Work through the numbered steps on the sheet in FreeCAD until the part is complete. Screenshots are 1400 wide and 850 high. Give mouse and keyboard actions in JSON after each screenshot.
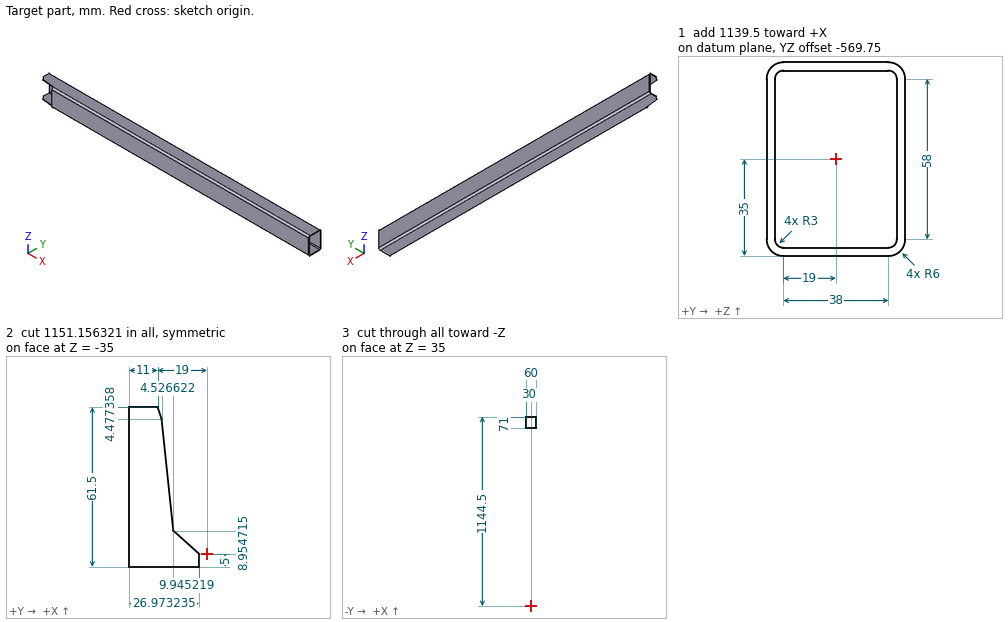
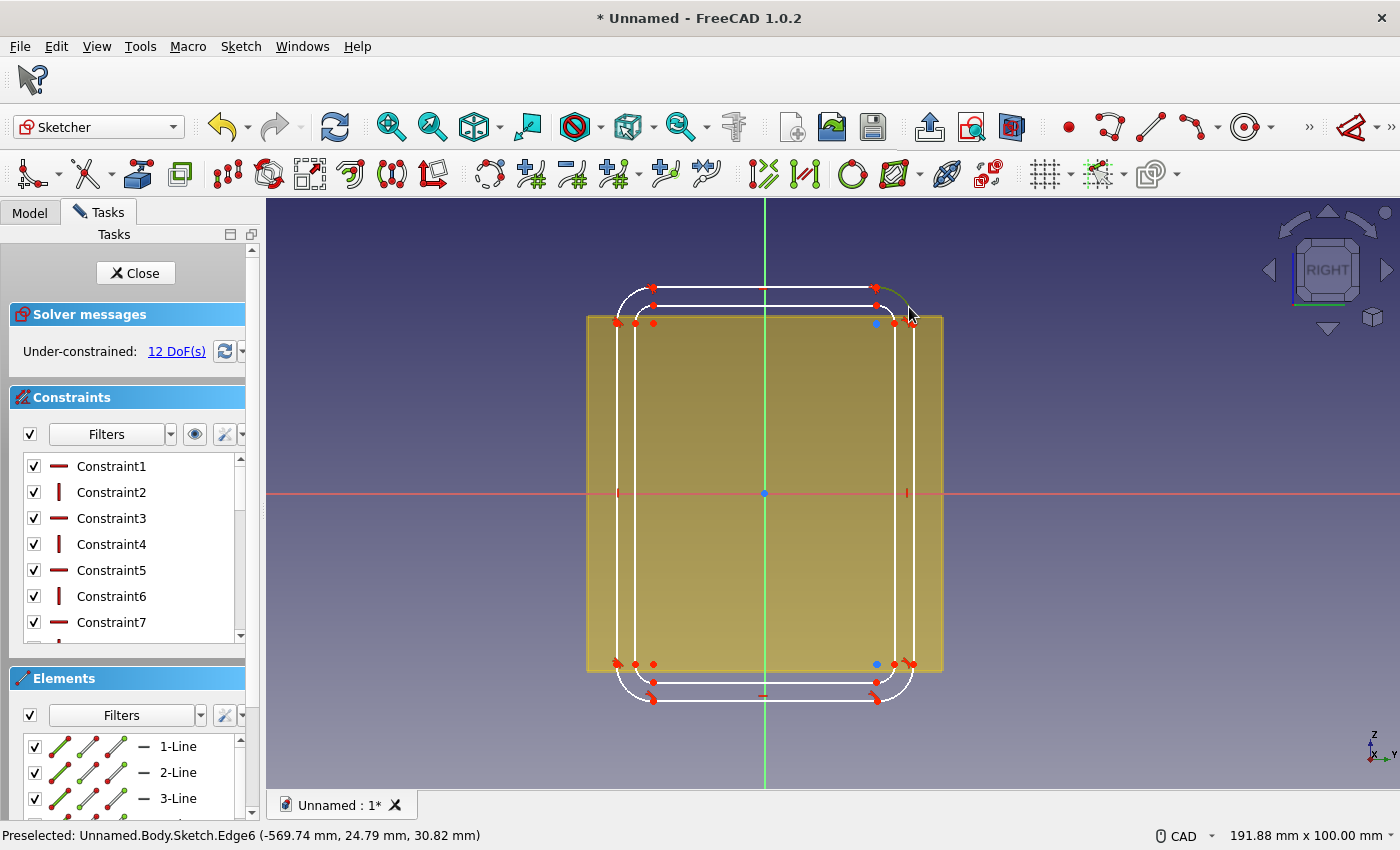
{"action": "left_click", "coordinate": [890, 311]}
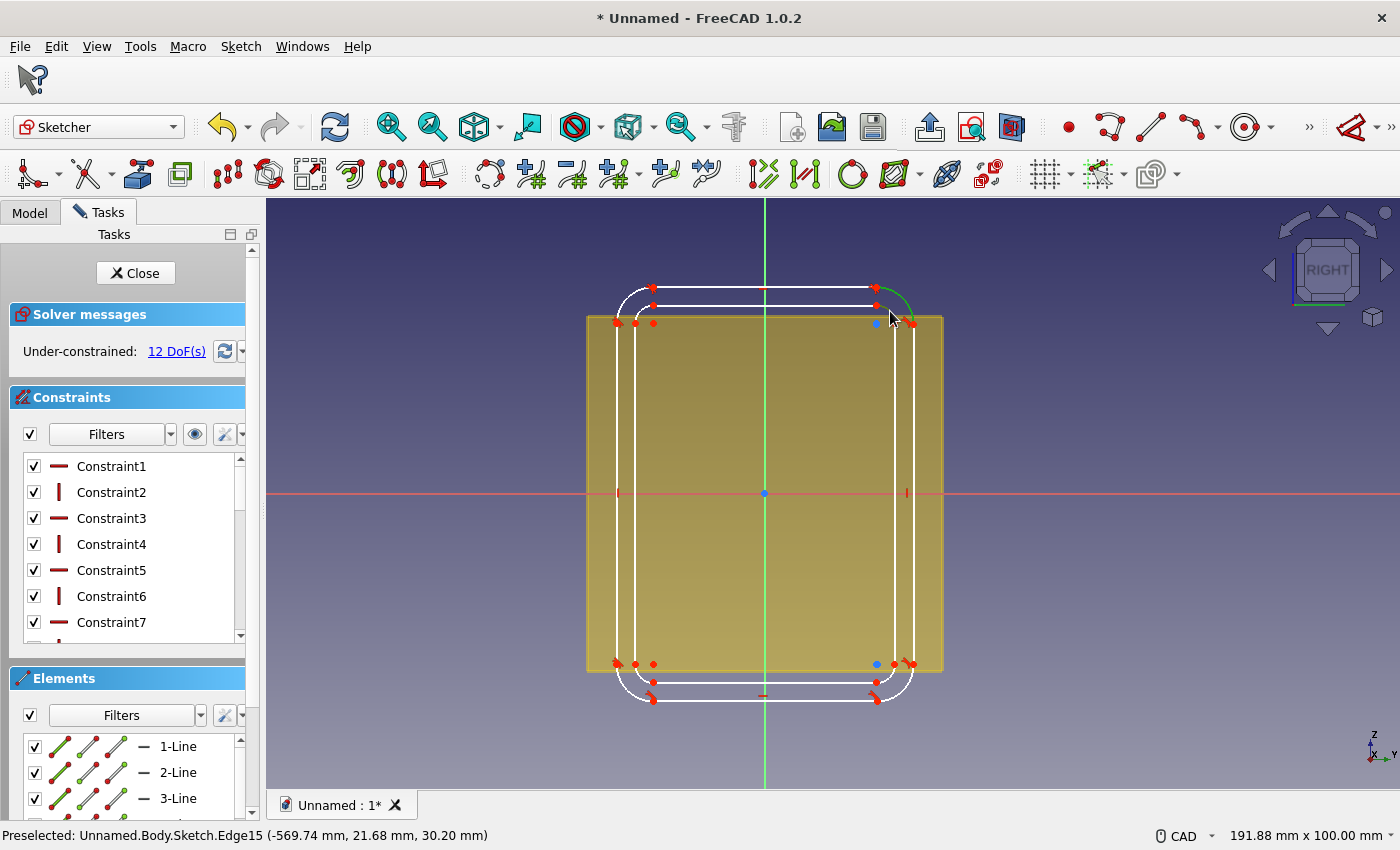
{"action": "key", "text": "c"}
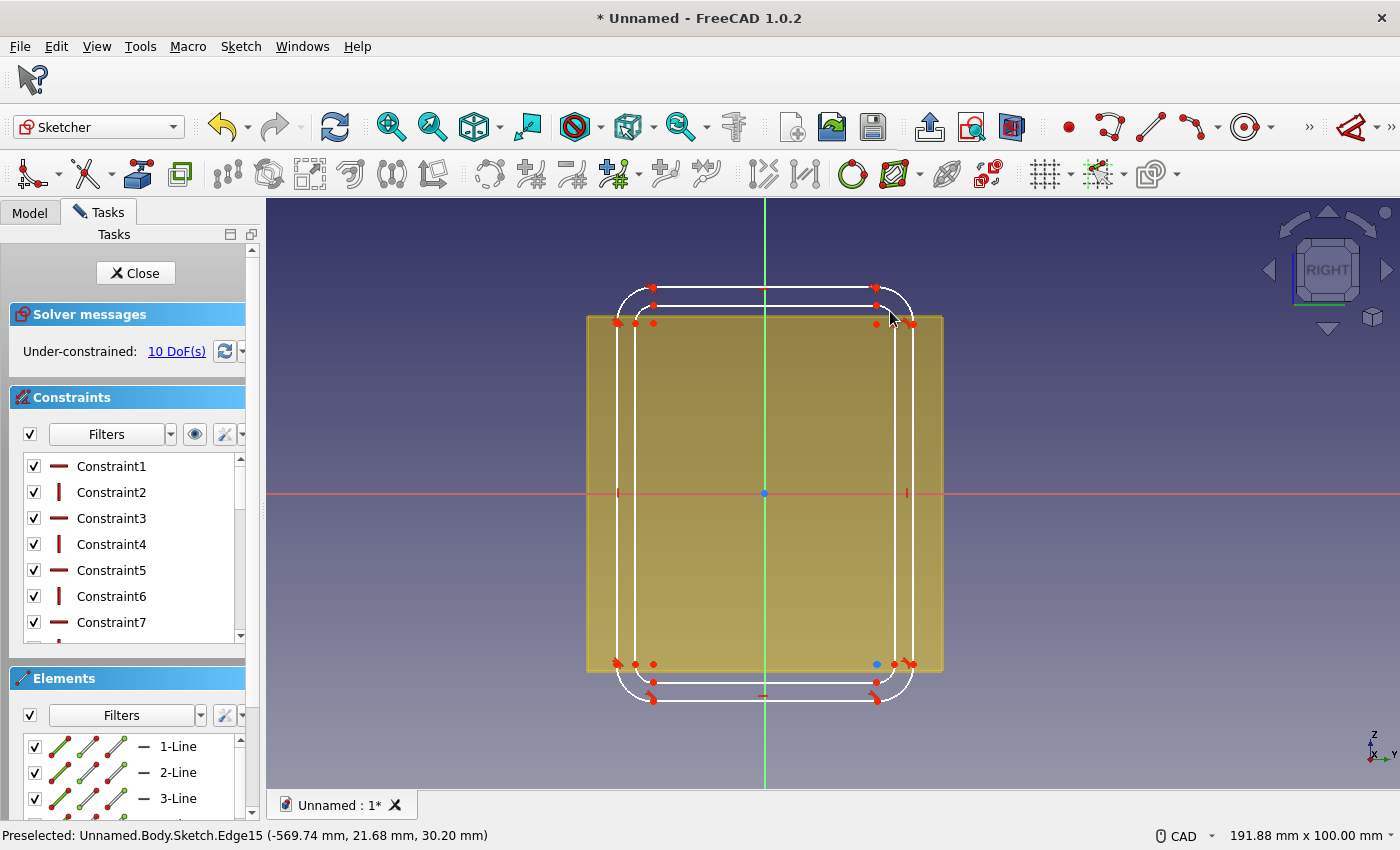
{"action": "left_click", "coordinate": [894, 697]}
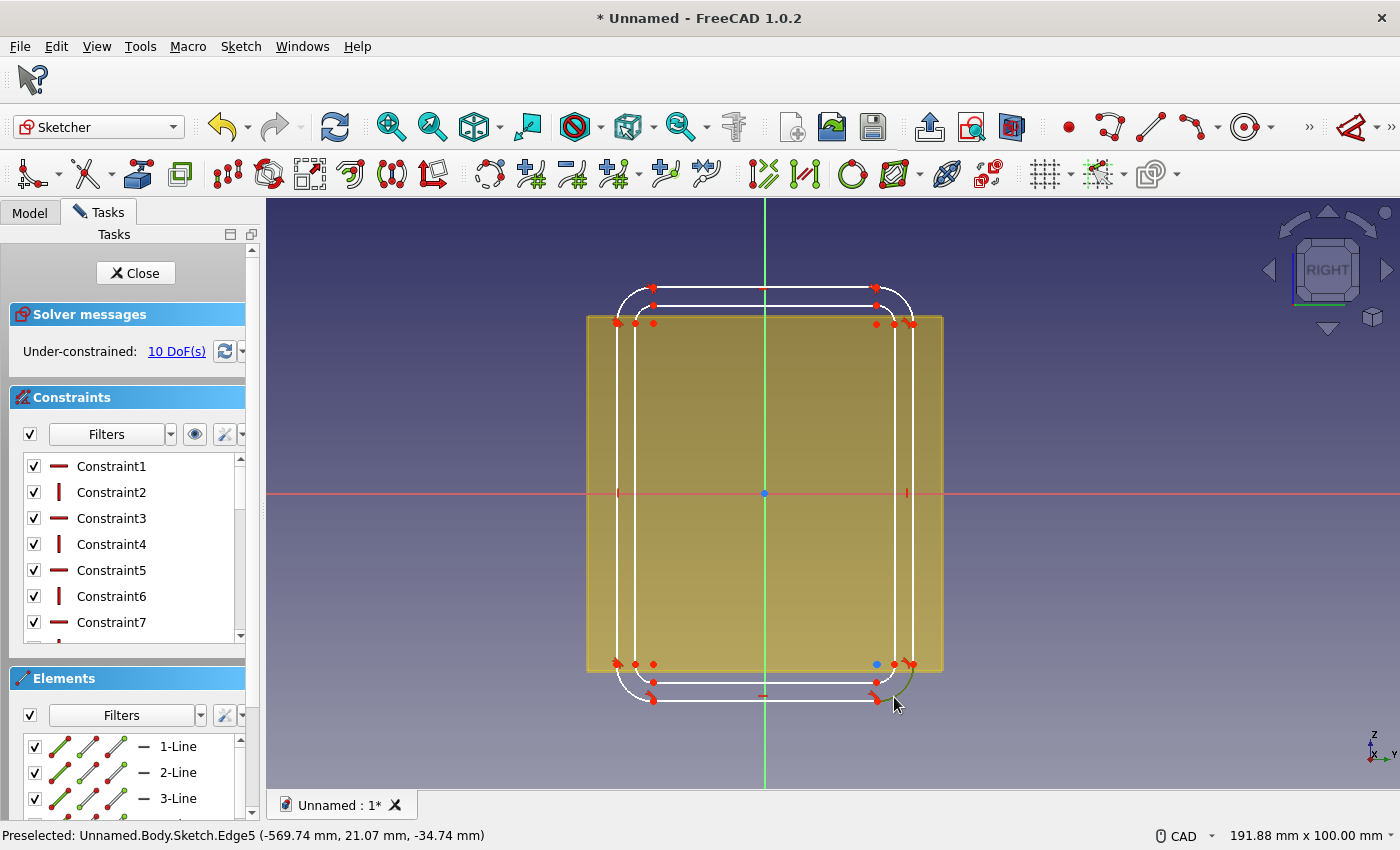
{"action": "left_click", "coordinate": [909, 307]}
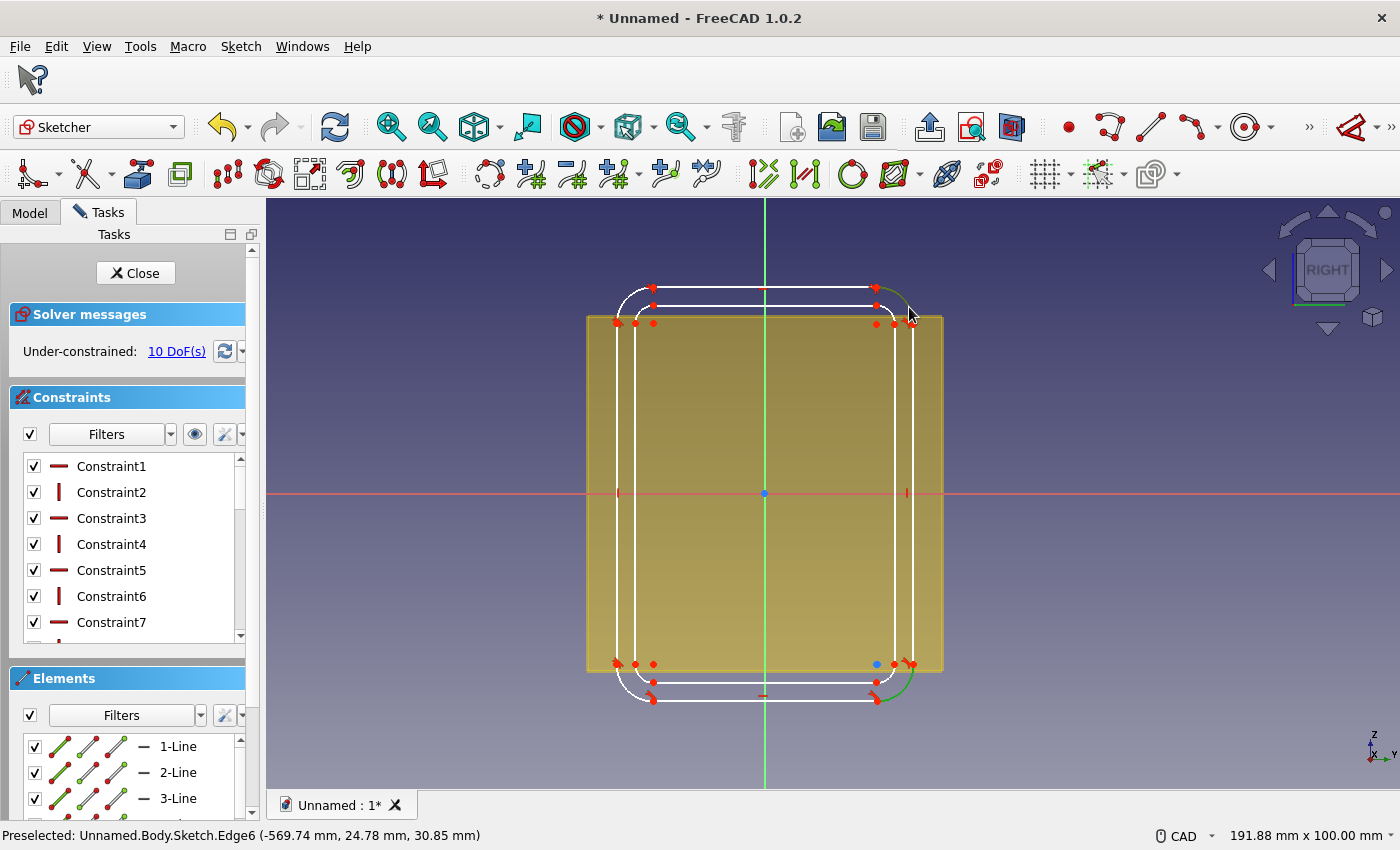
{"action": "left_click", "coordinate": [637, 291]}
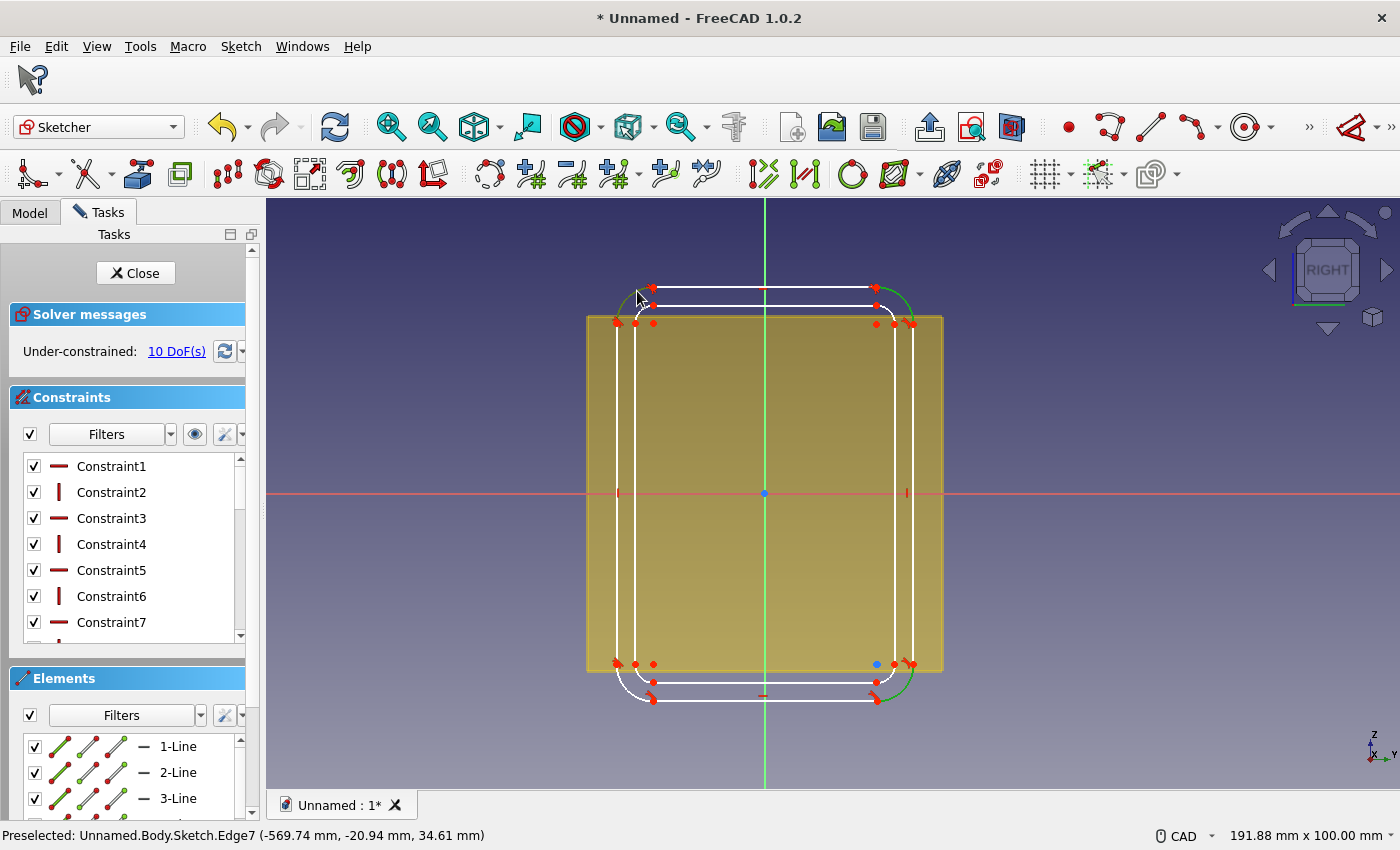
{"action": "left_click", "coordinate": [621, 681]}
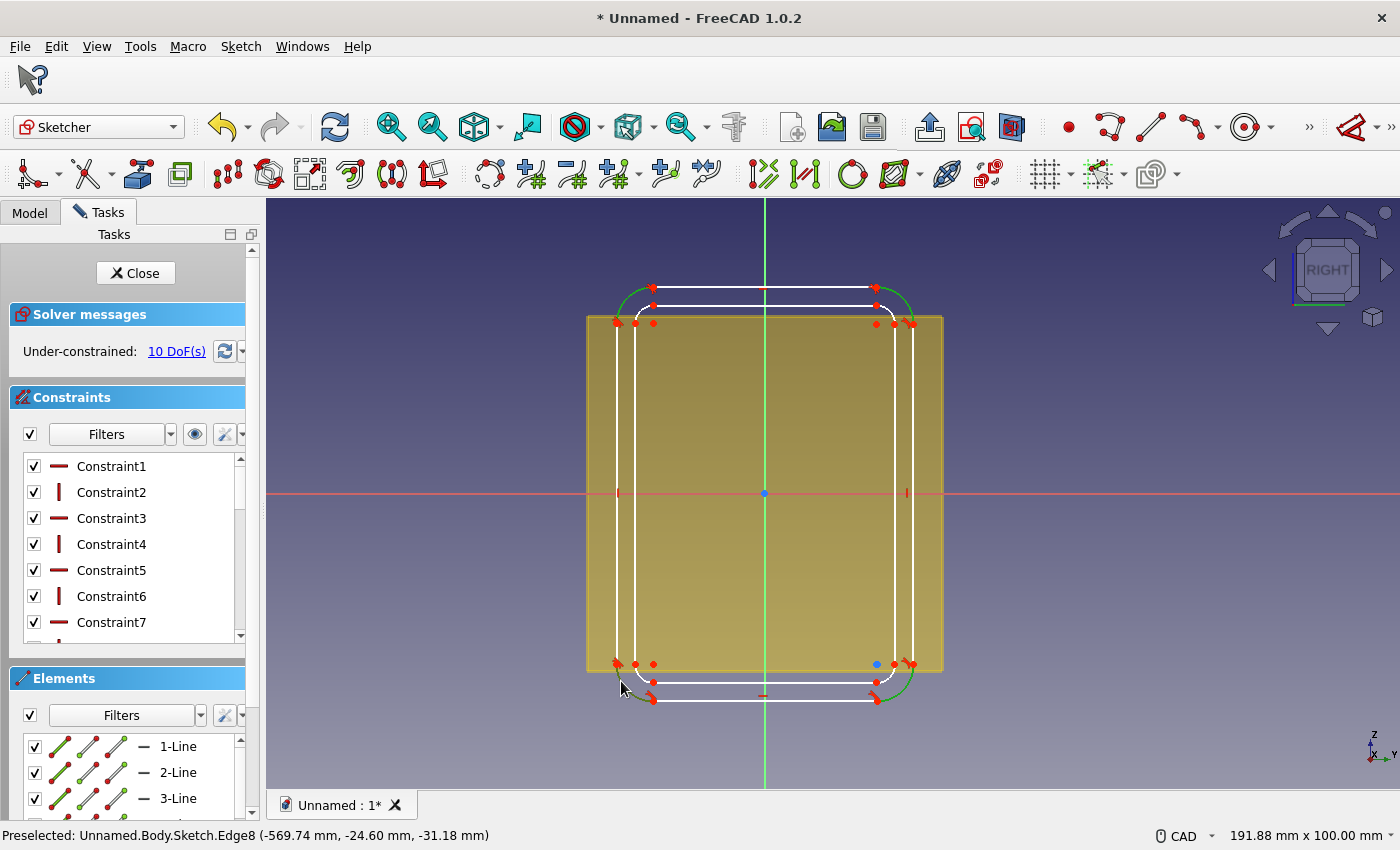
{"action": "key", "text": "e"}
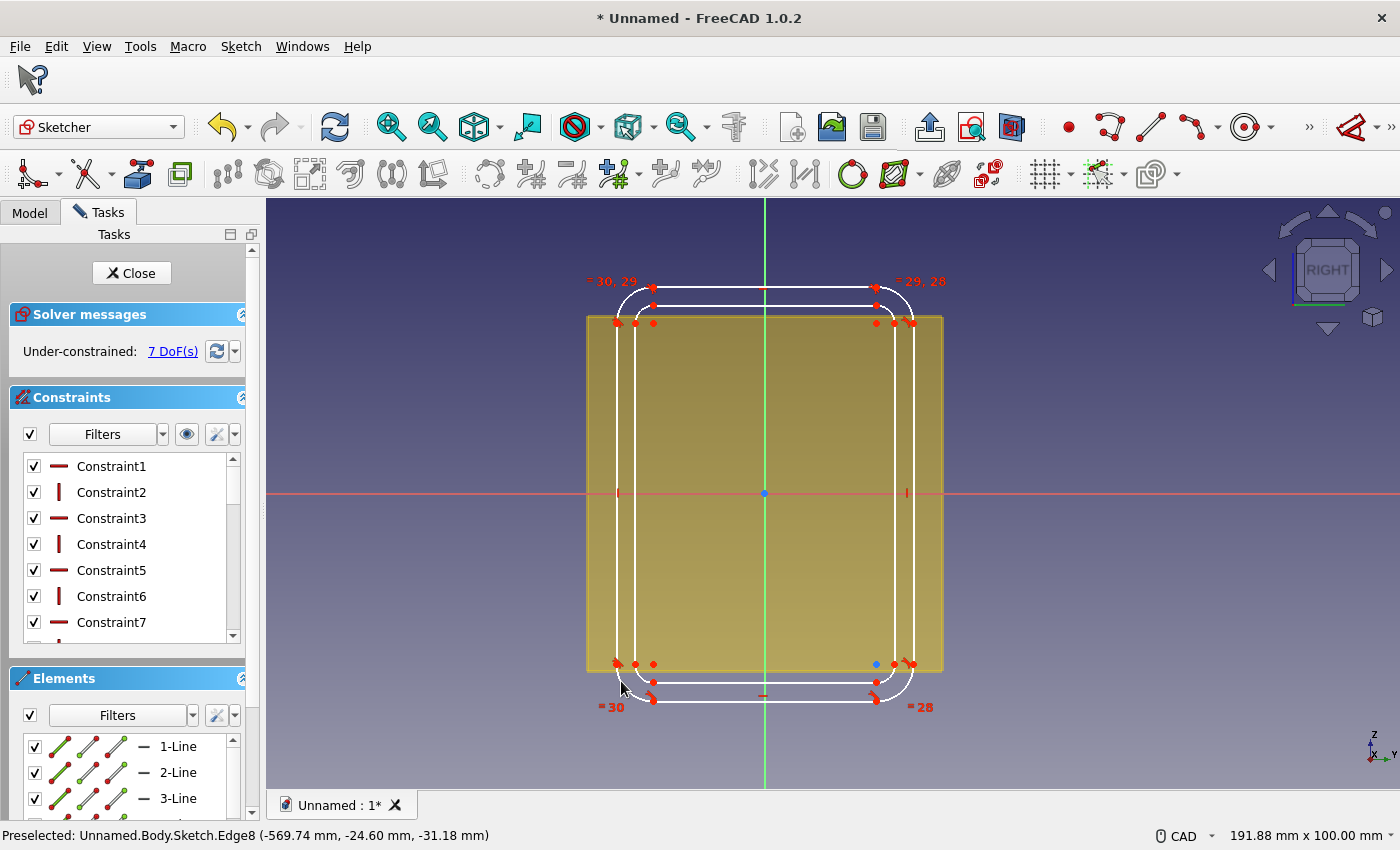
{"action": "left_click", "coordinate": [641, 678]}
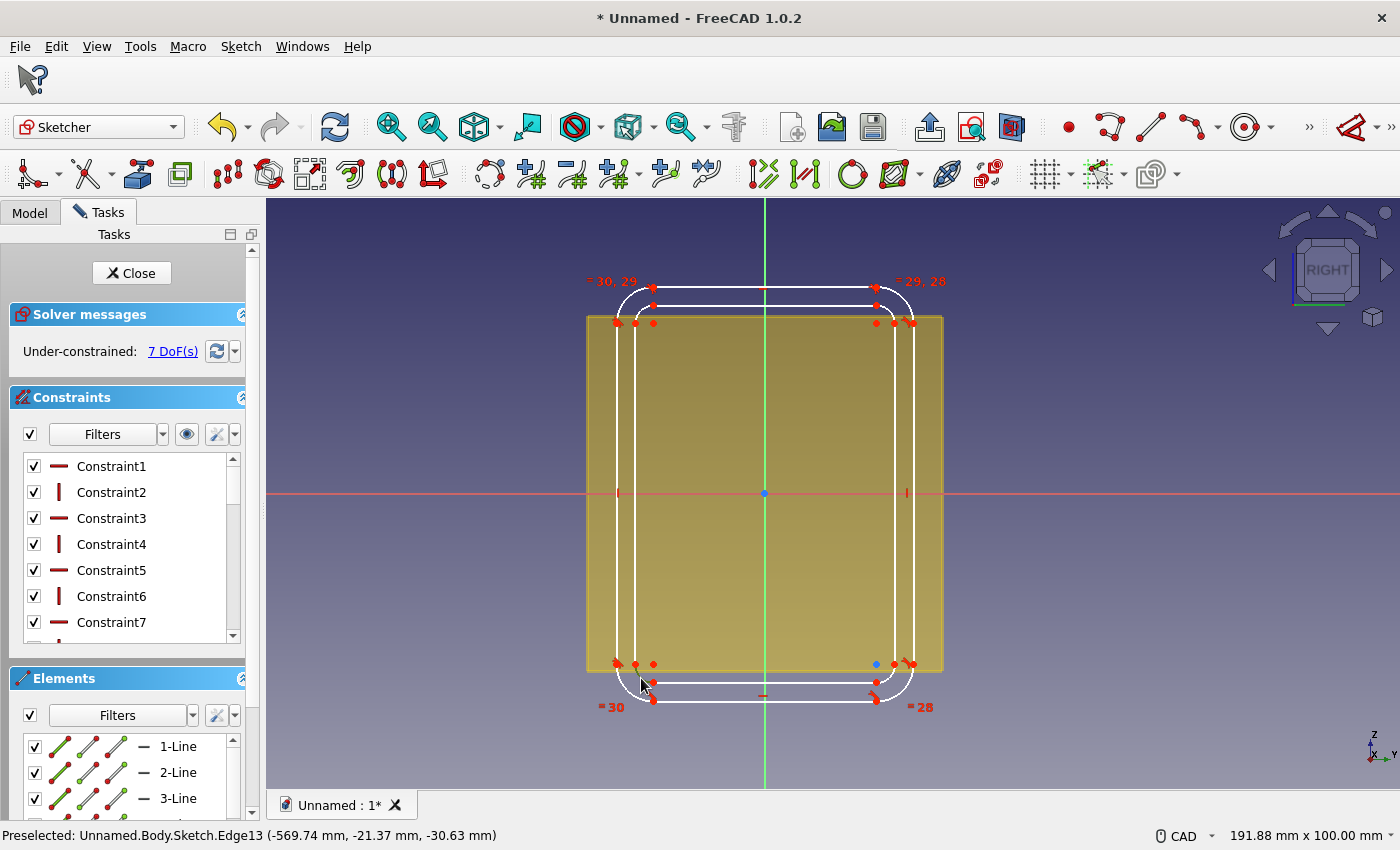
{"action": "left_click", "coordinate": [890, 678]}